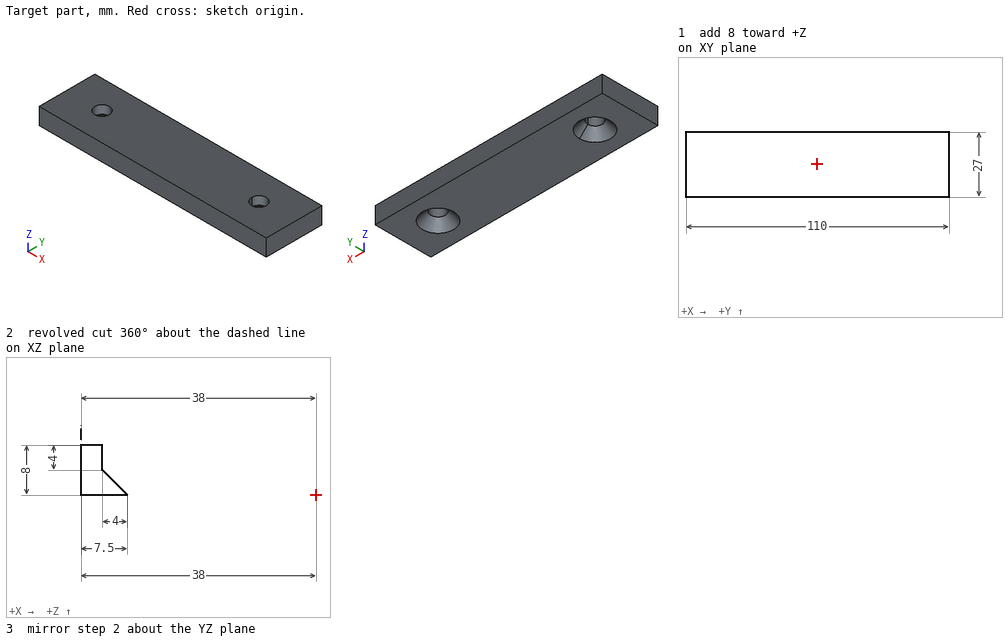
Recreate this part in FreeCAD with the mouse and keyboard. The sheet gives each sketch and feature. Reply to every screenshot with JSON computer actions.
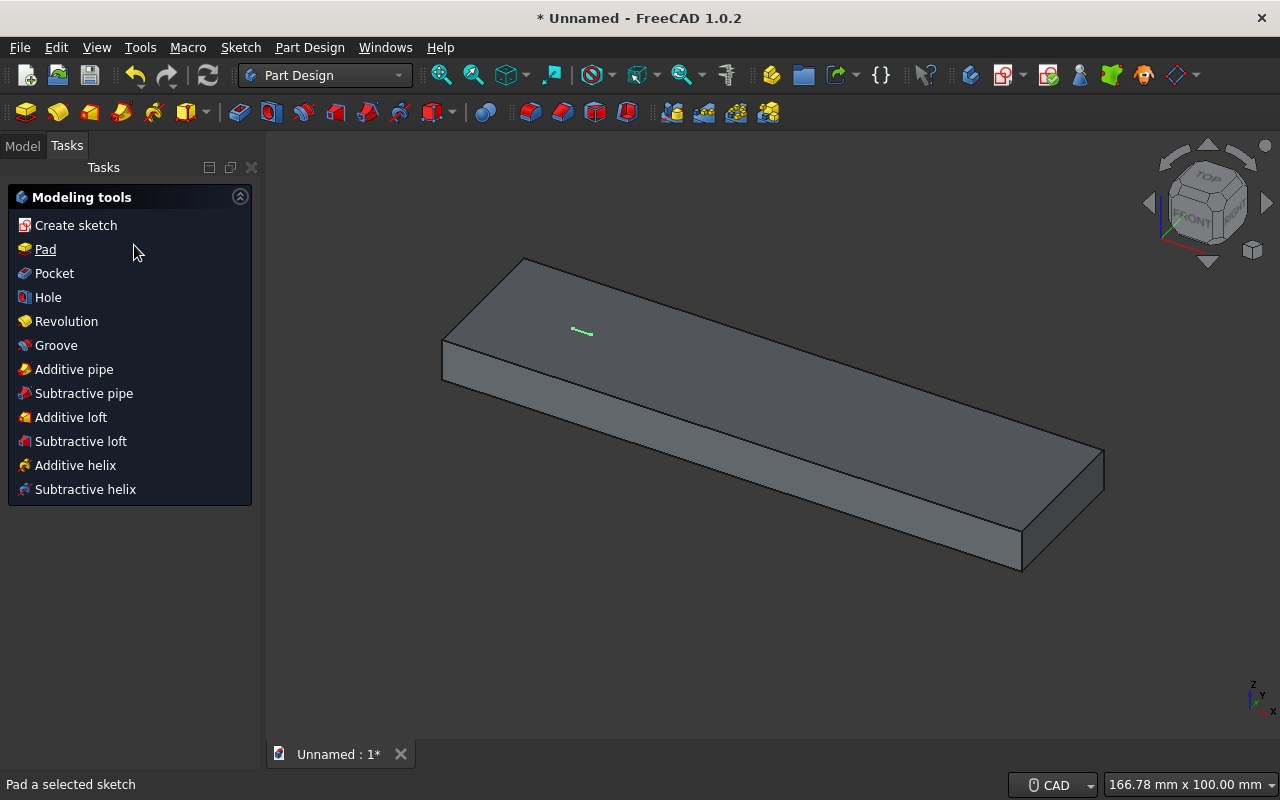
{"action": "left_click", "coordinate": [304, 112]}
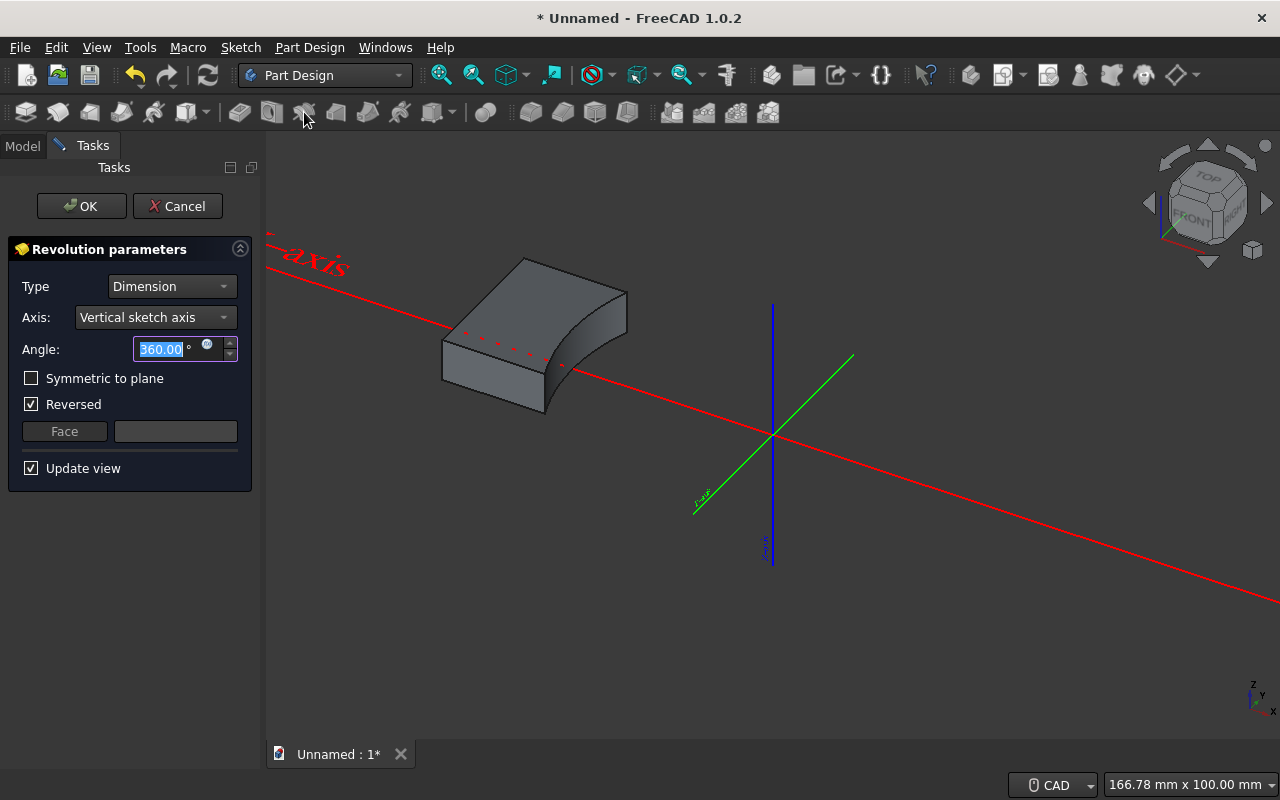
{"action": "left_click", "coordinate": [156, 318]}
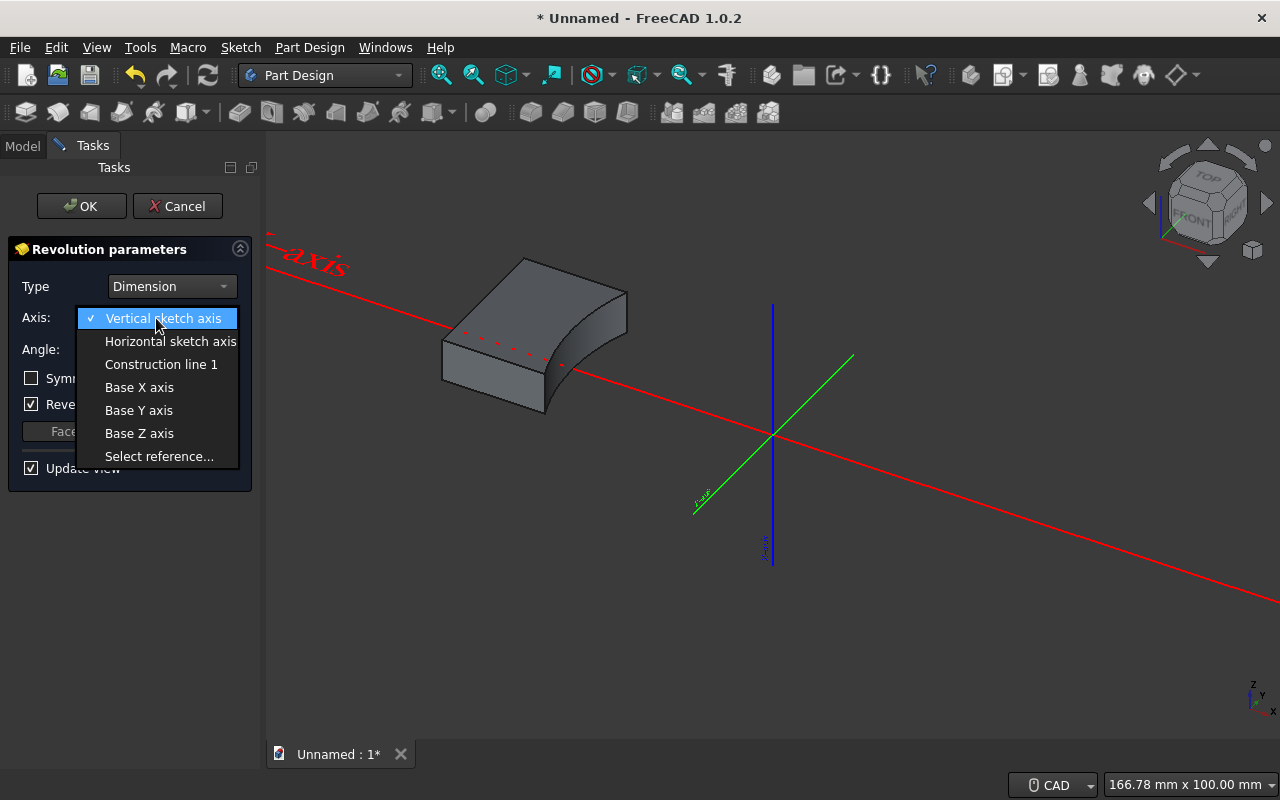
{"action": "left_click", "coordinate": [156, 364]}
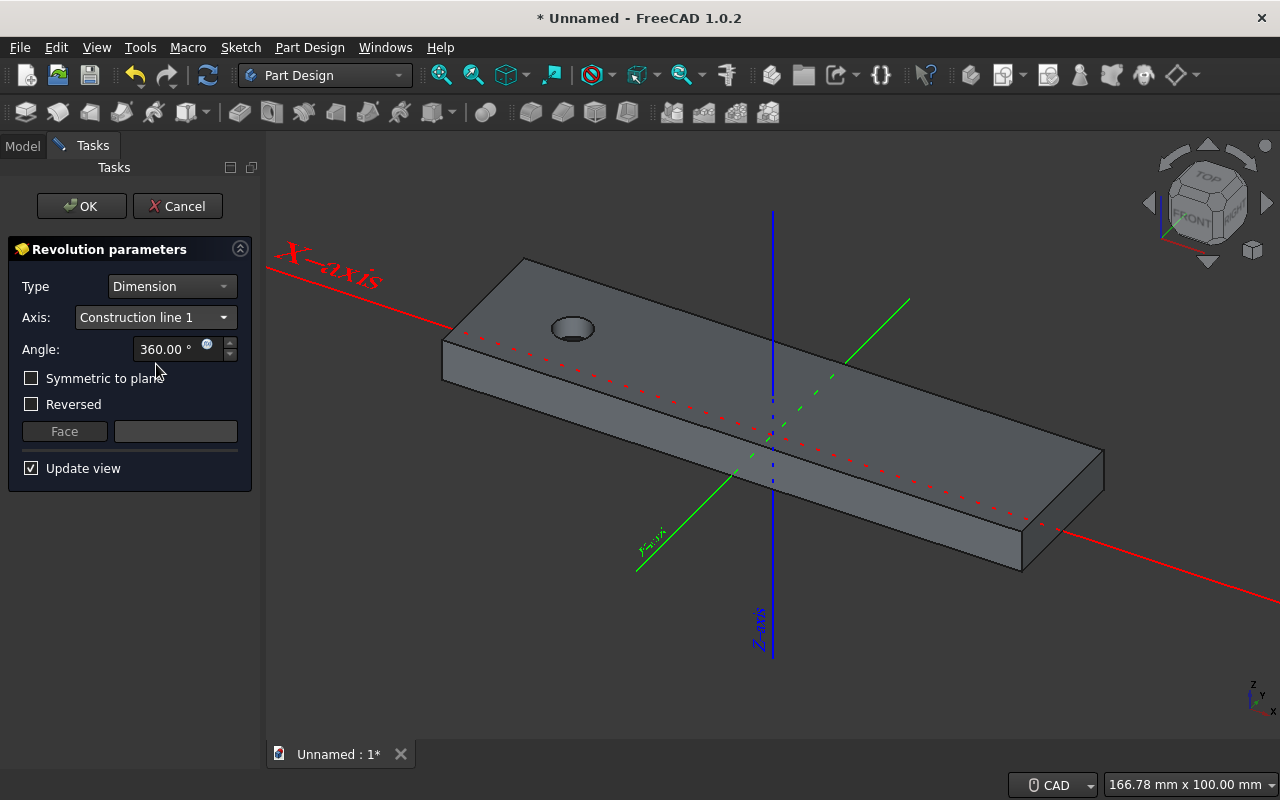
{"action": "left_click", "coordinate": [82, 206]}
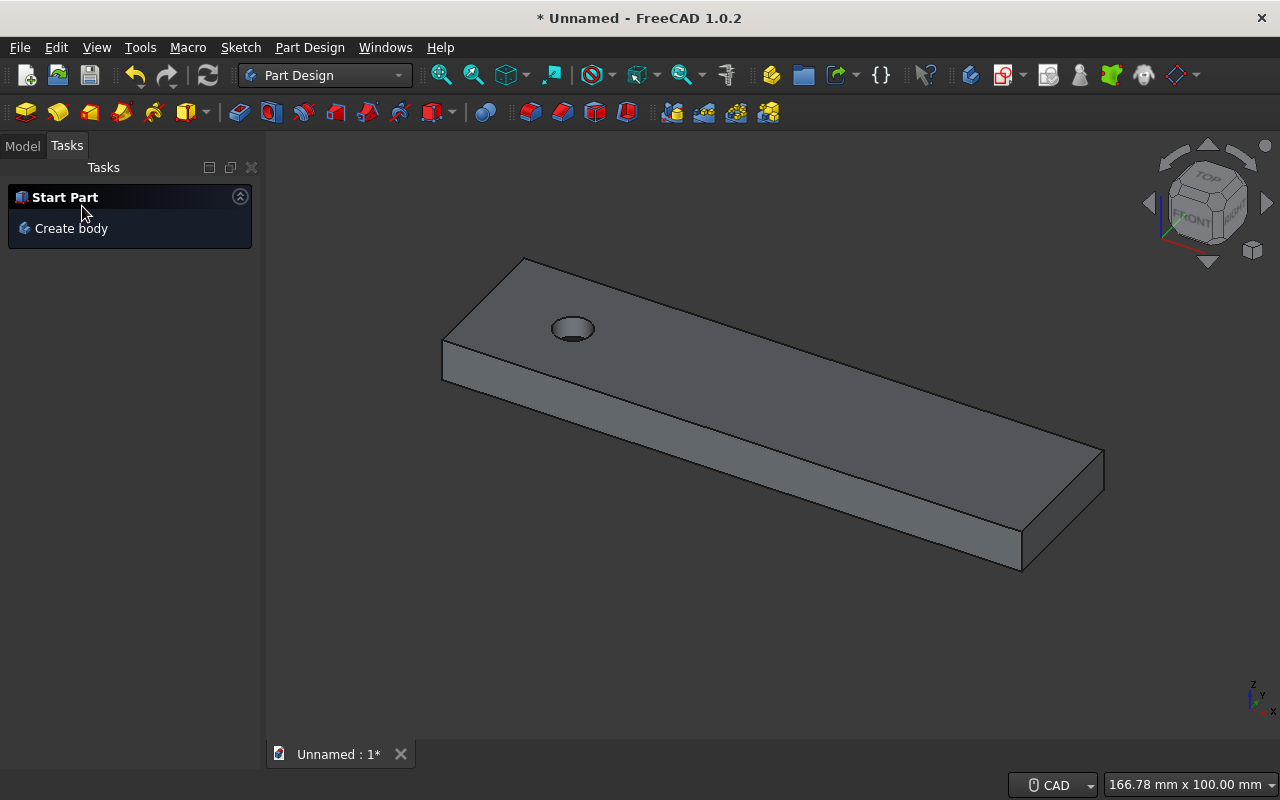
{"action": "left_click", "coordinate": [23, 145]}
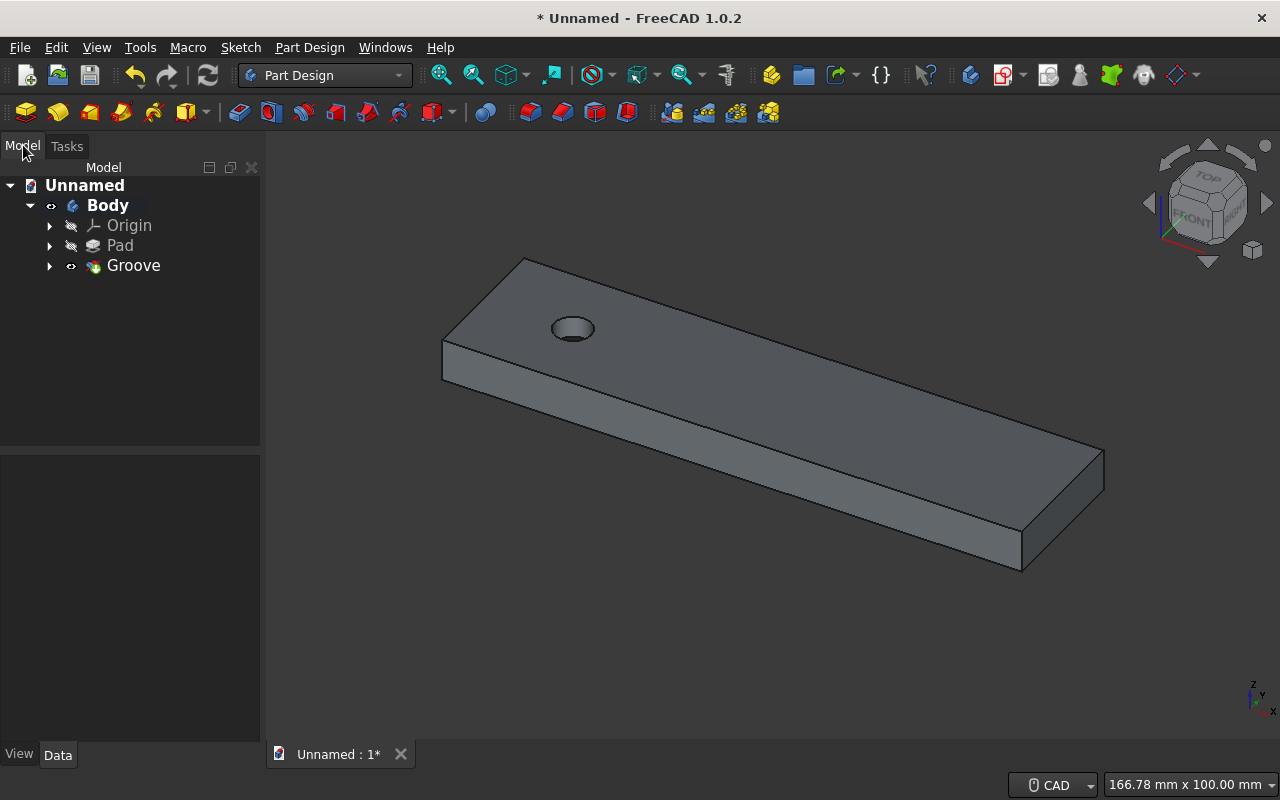
{"action": "left_click", "coordinate": [116, 266]}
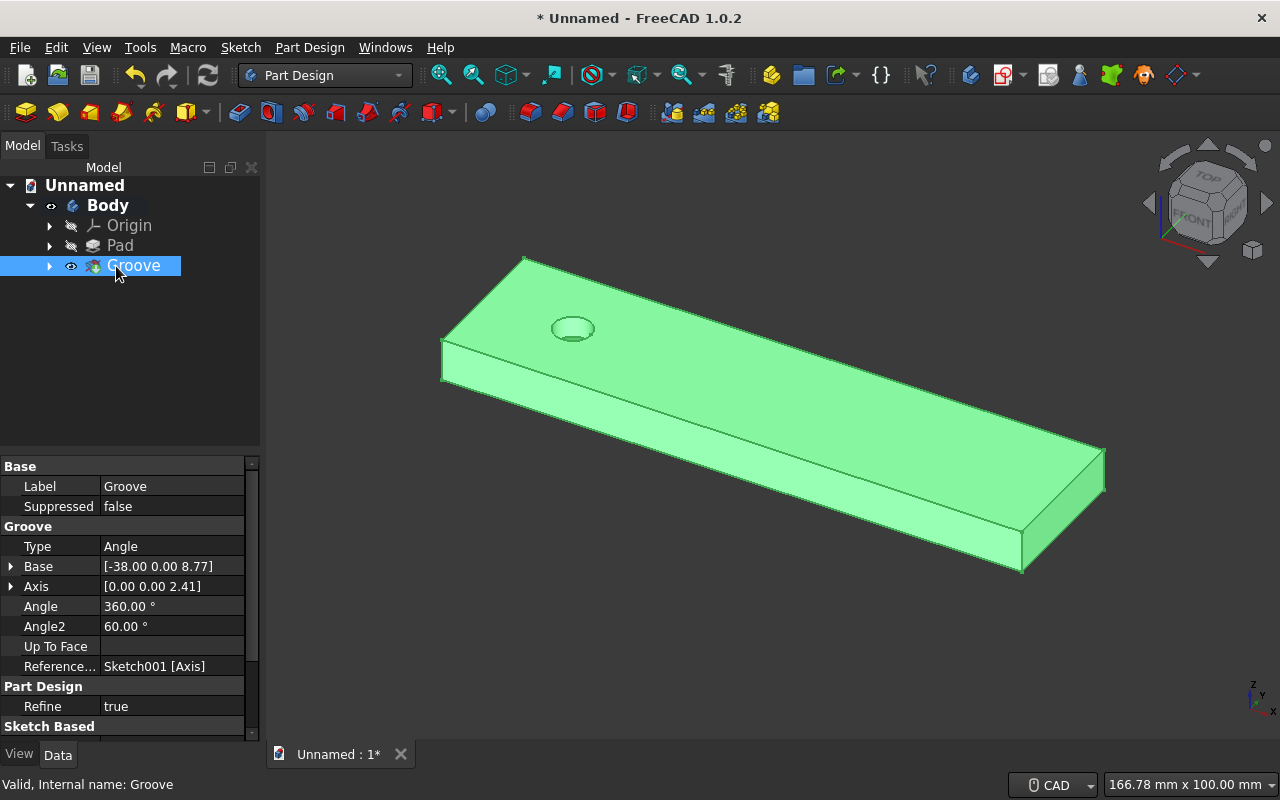
{"action": "left_click", "coordinate": [672, 112]}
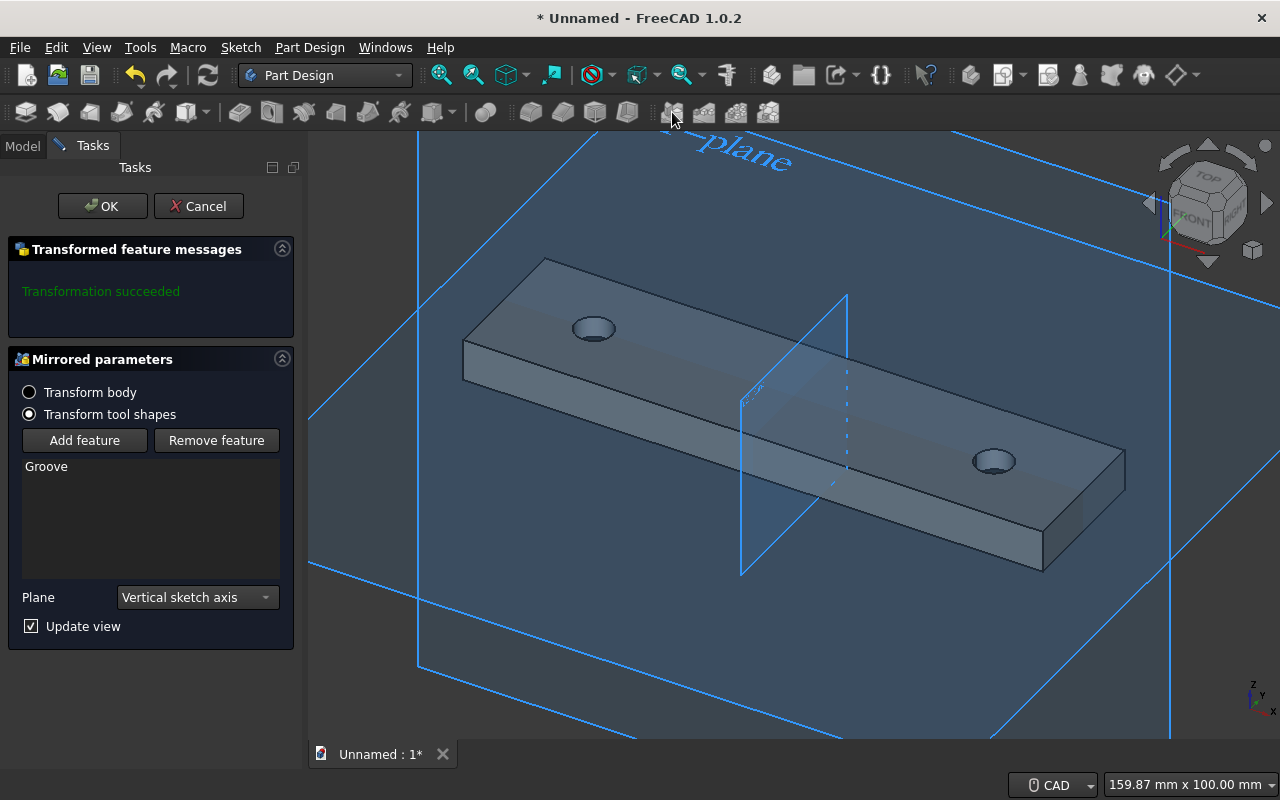
{"action": "left_click", "coordinate": [198, 598]}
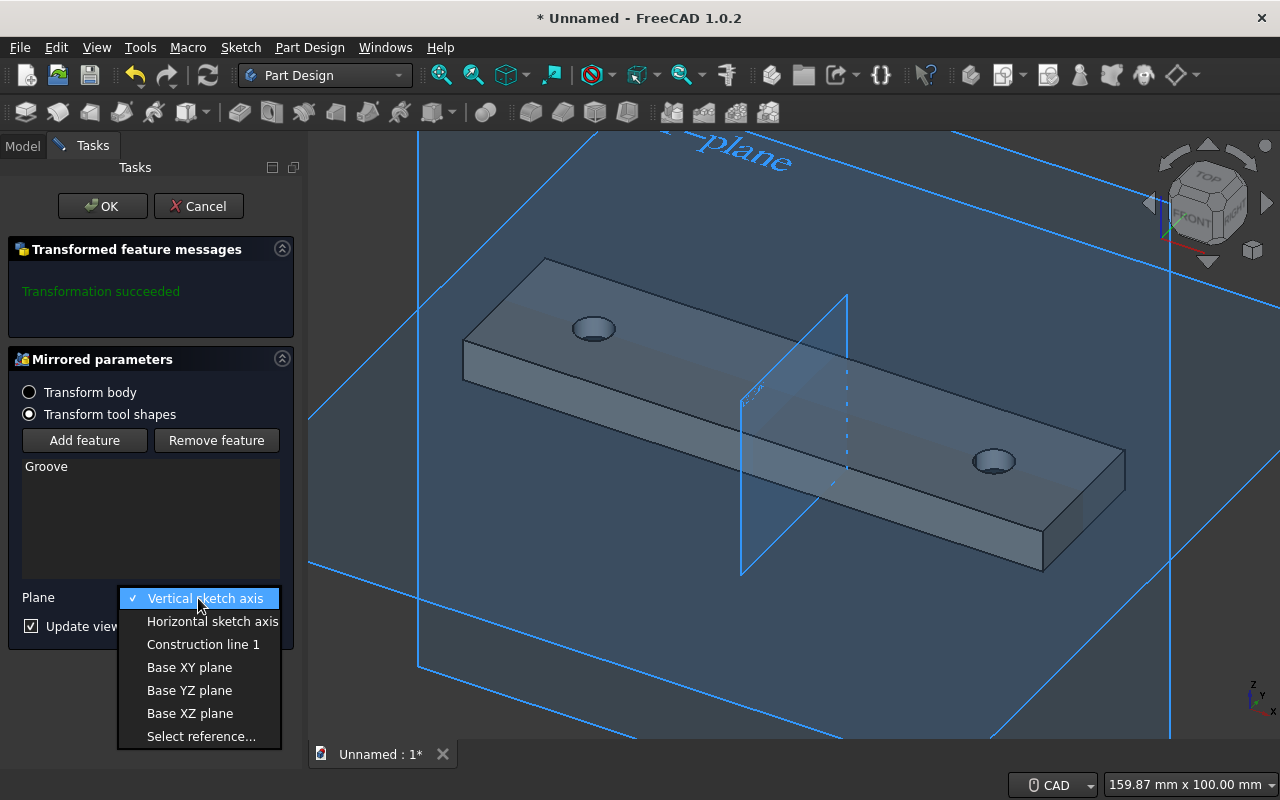
{"action": "left_click", "coordinate": [198, 690]}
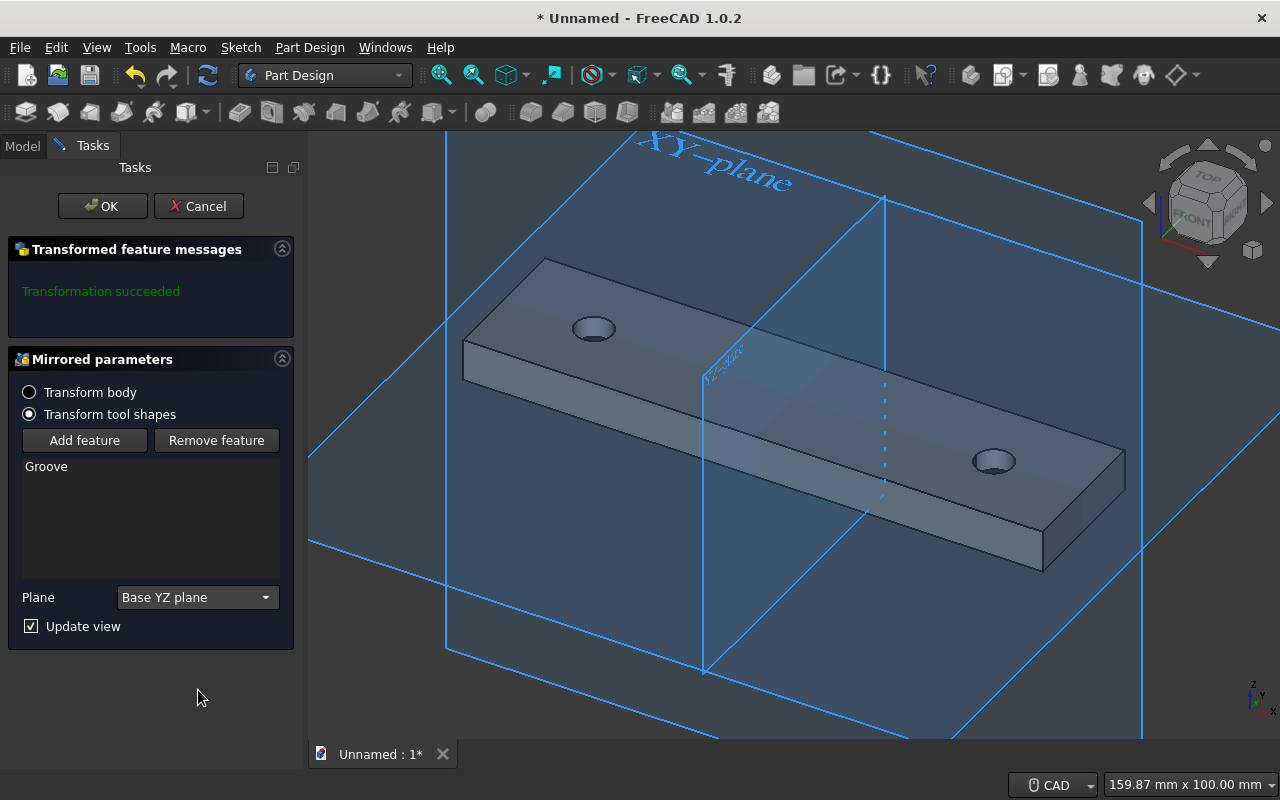
{"action": "left_click", "coordinate": [103, 206]}